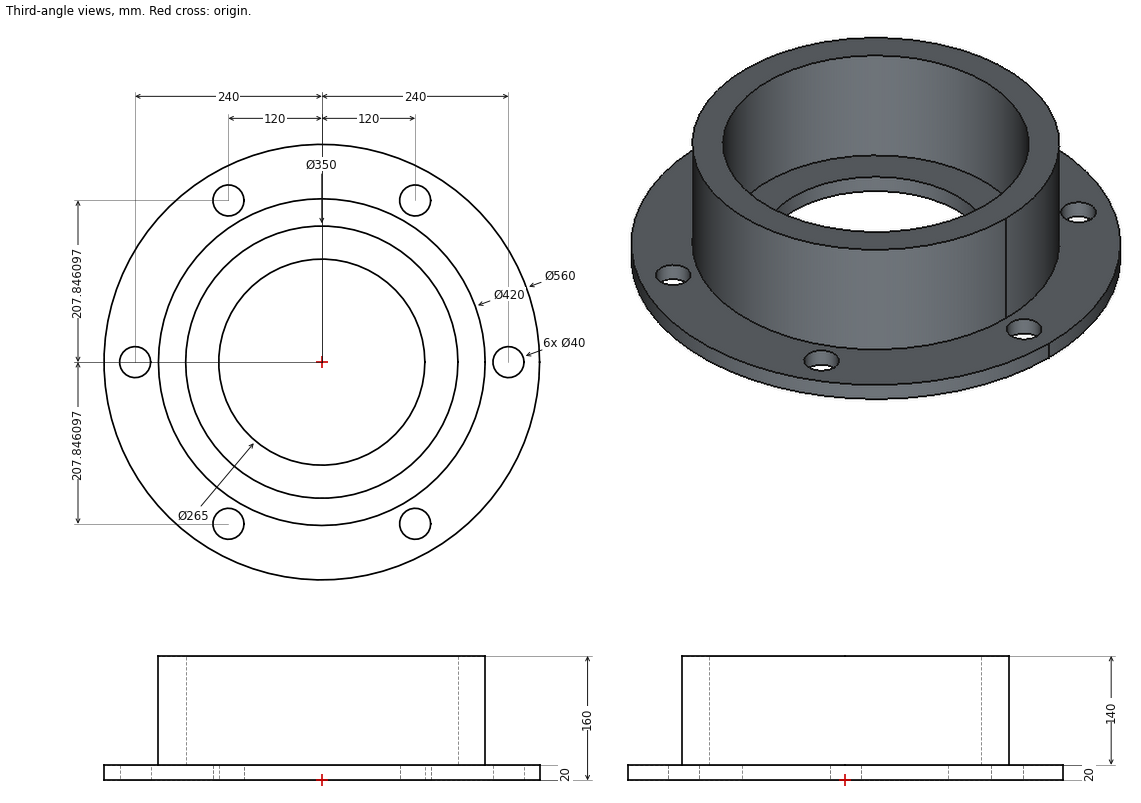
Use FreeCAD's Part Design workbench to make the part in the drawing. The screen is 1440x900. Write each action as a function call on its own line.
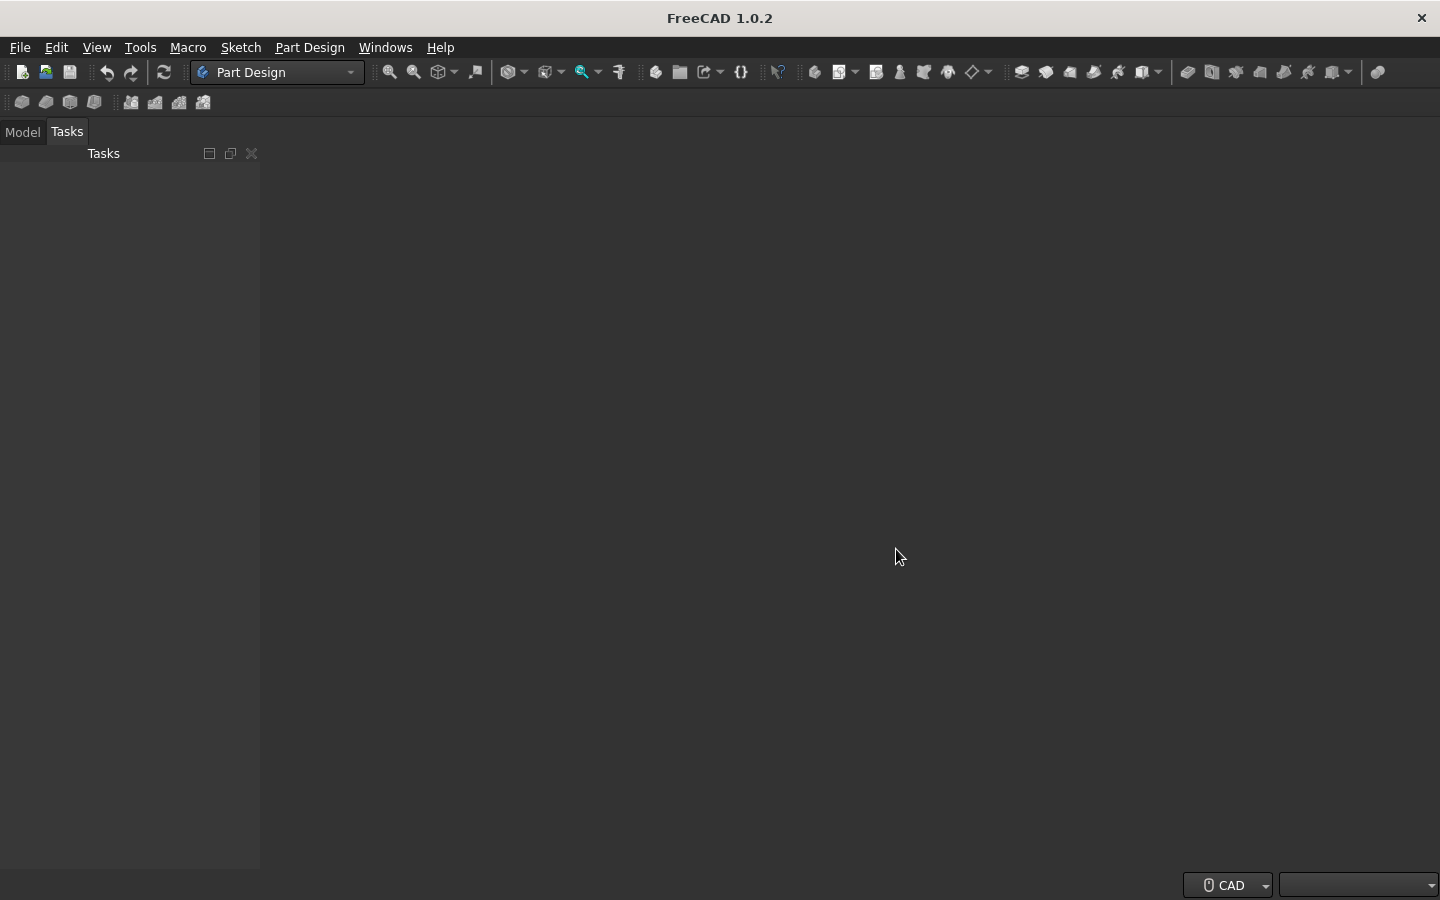
click(22, 72)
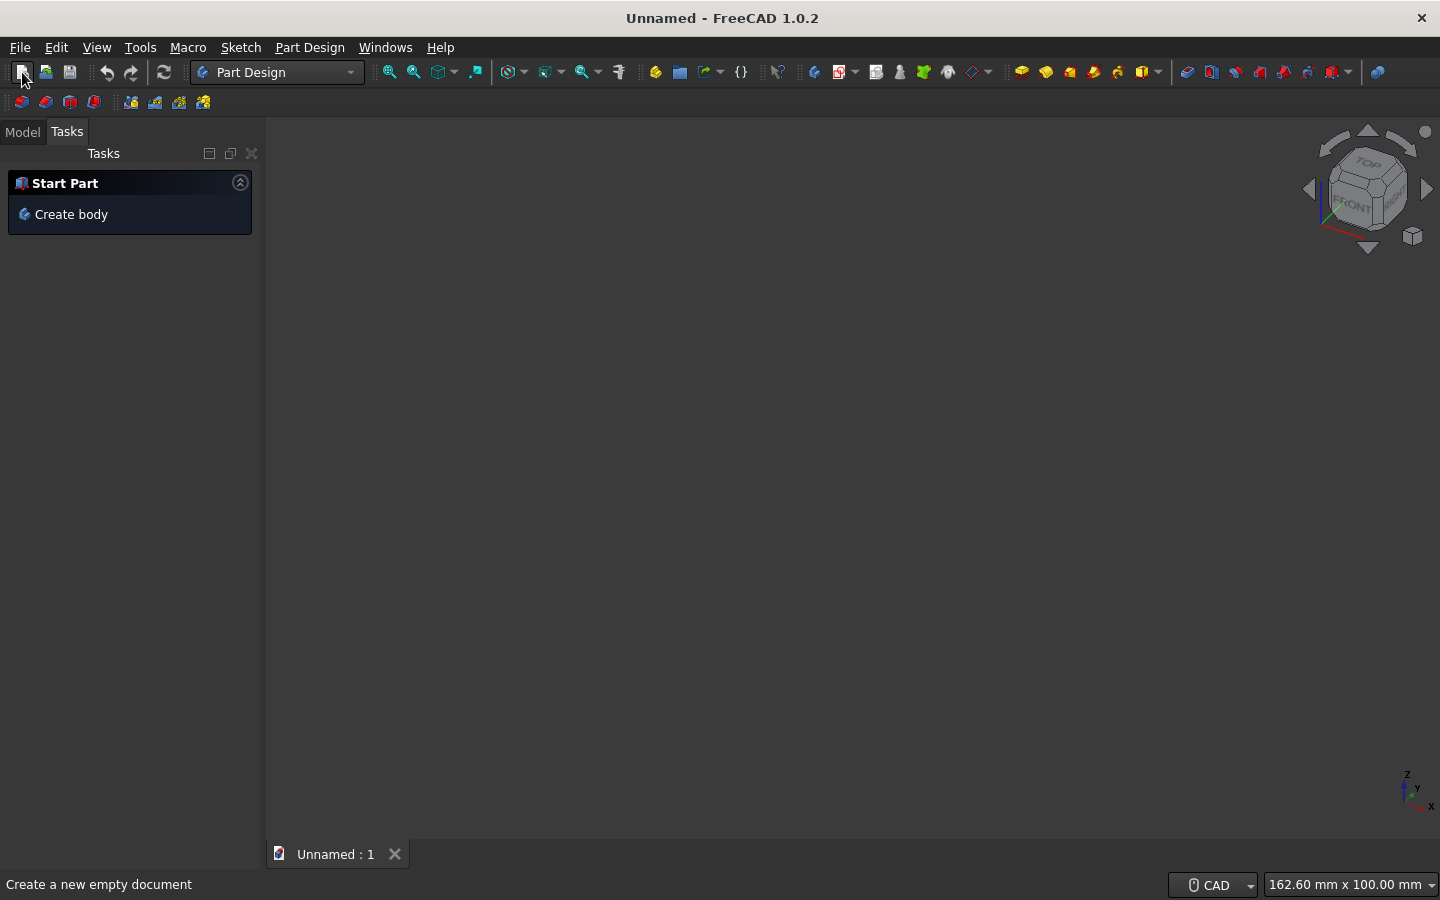
click(840, 72)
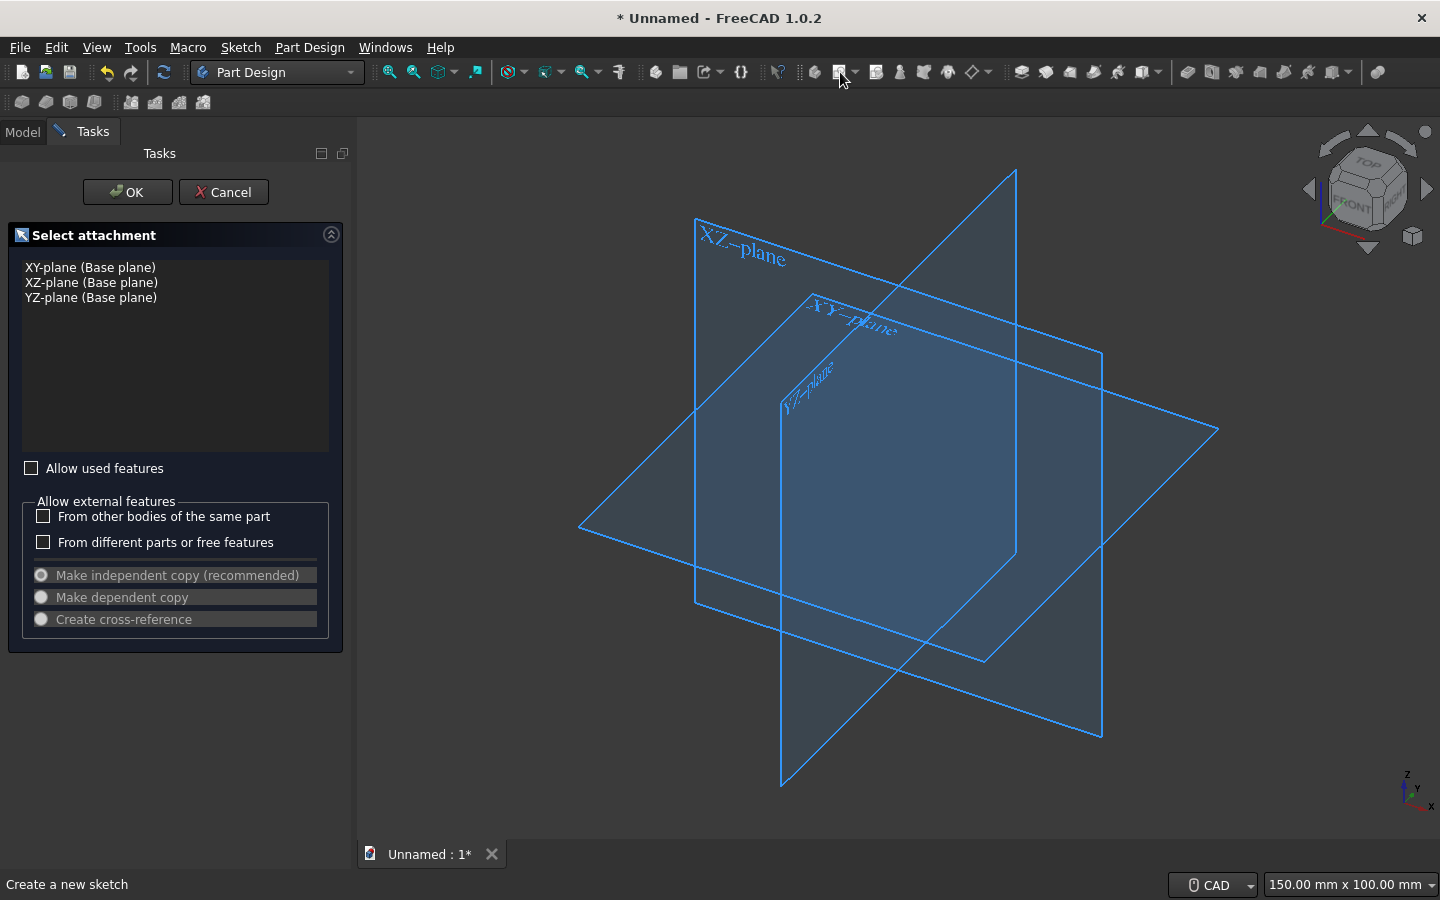
click(82, 268)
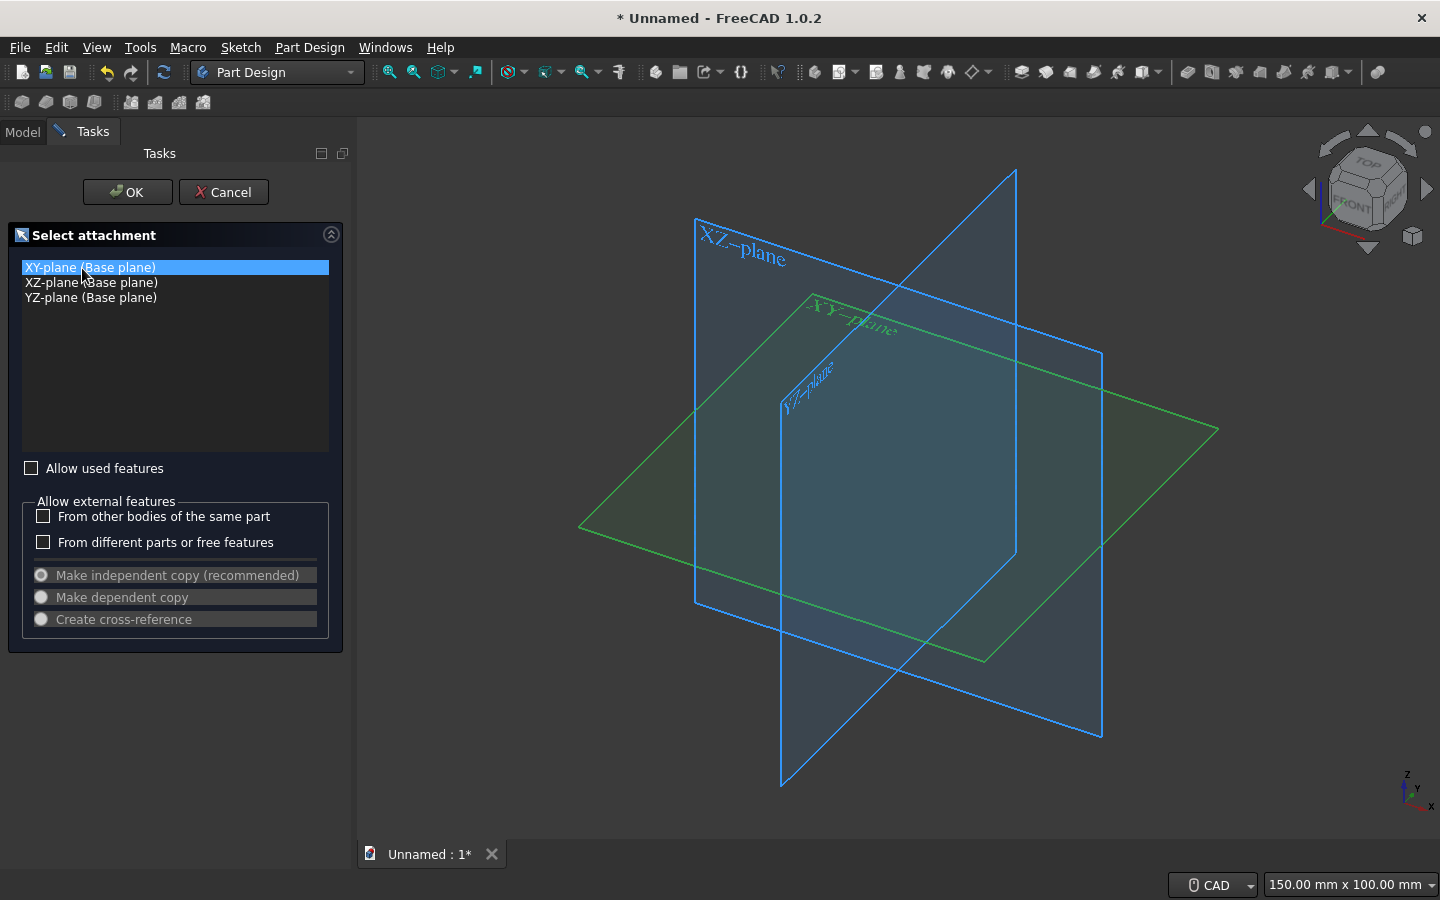
click(128, 192)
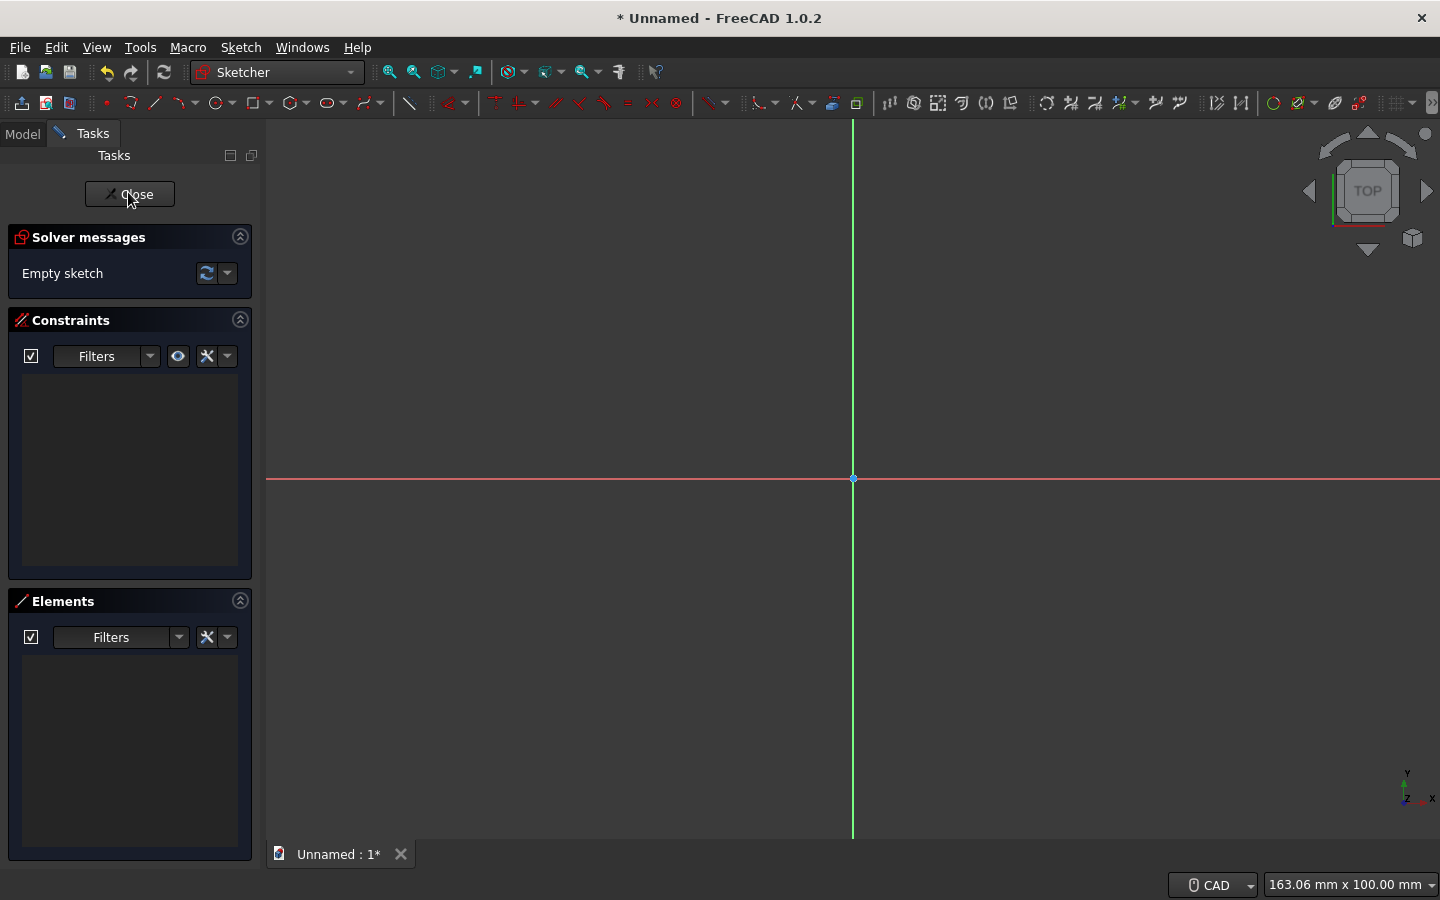
scroll(776, 479, down, 11)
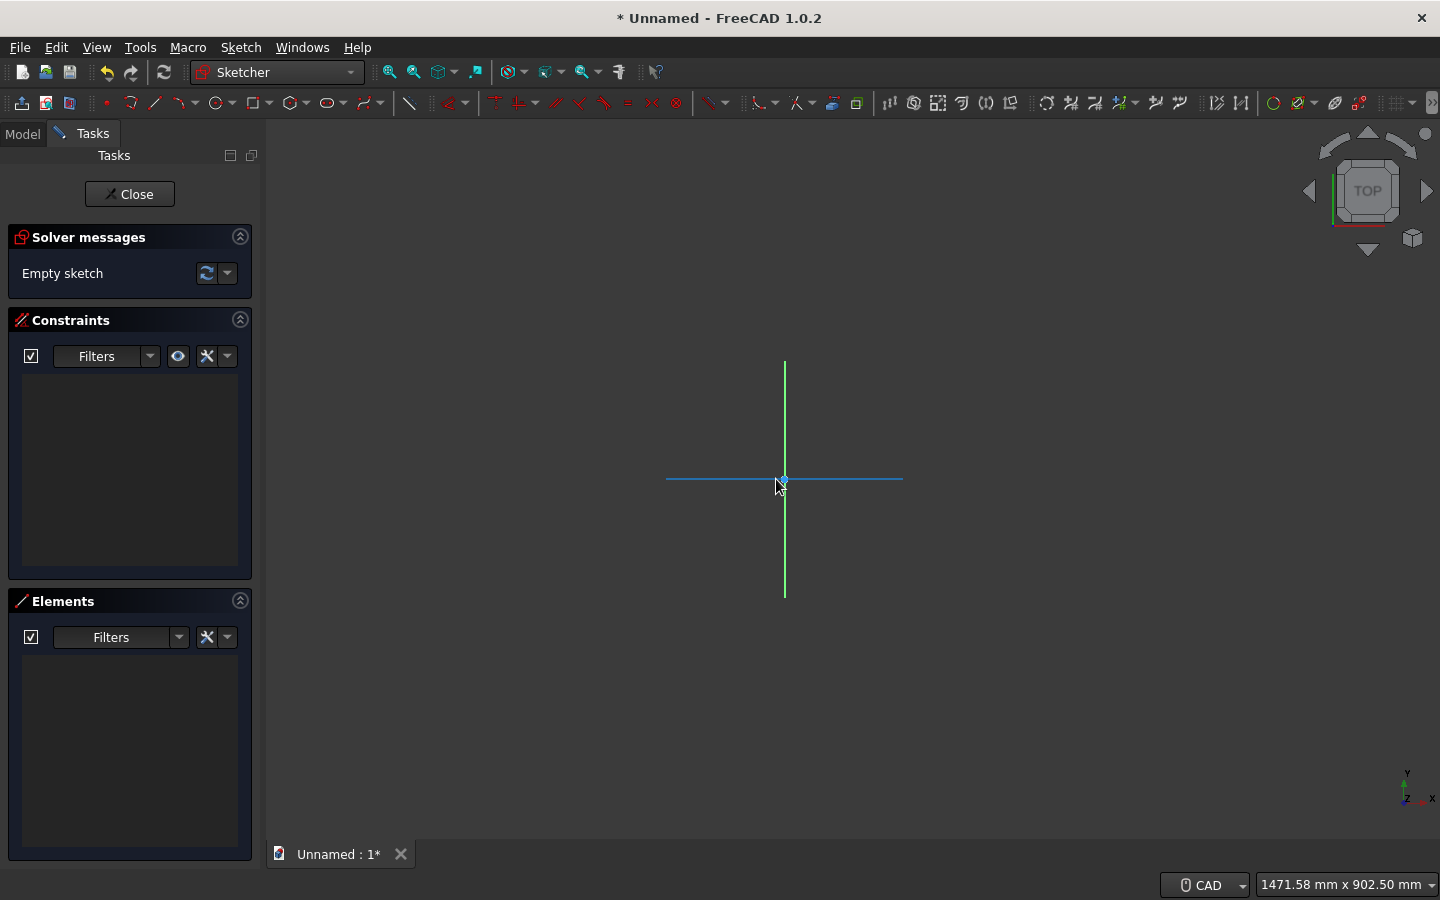
key(g)
key(c)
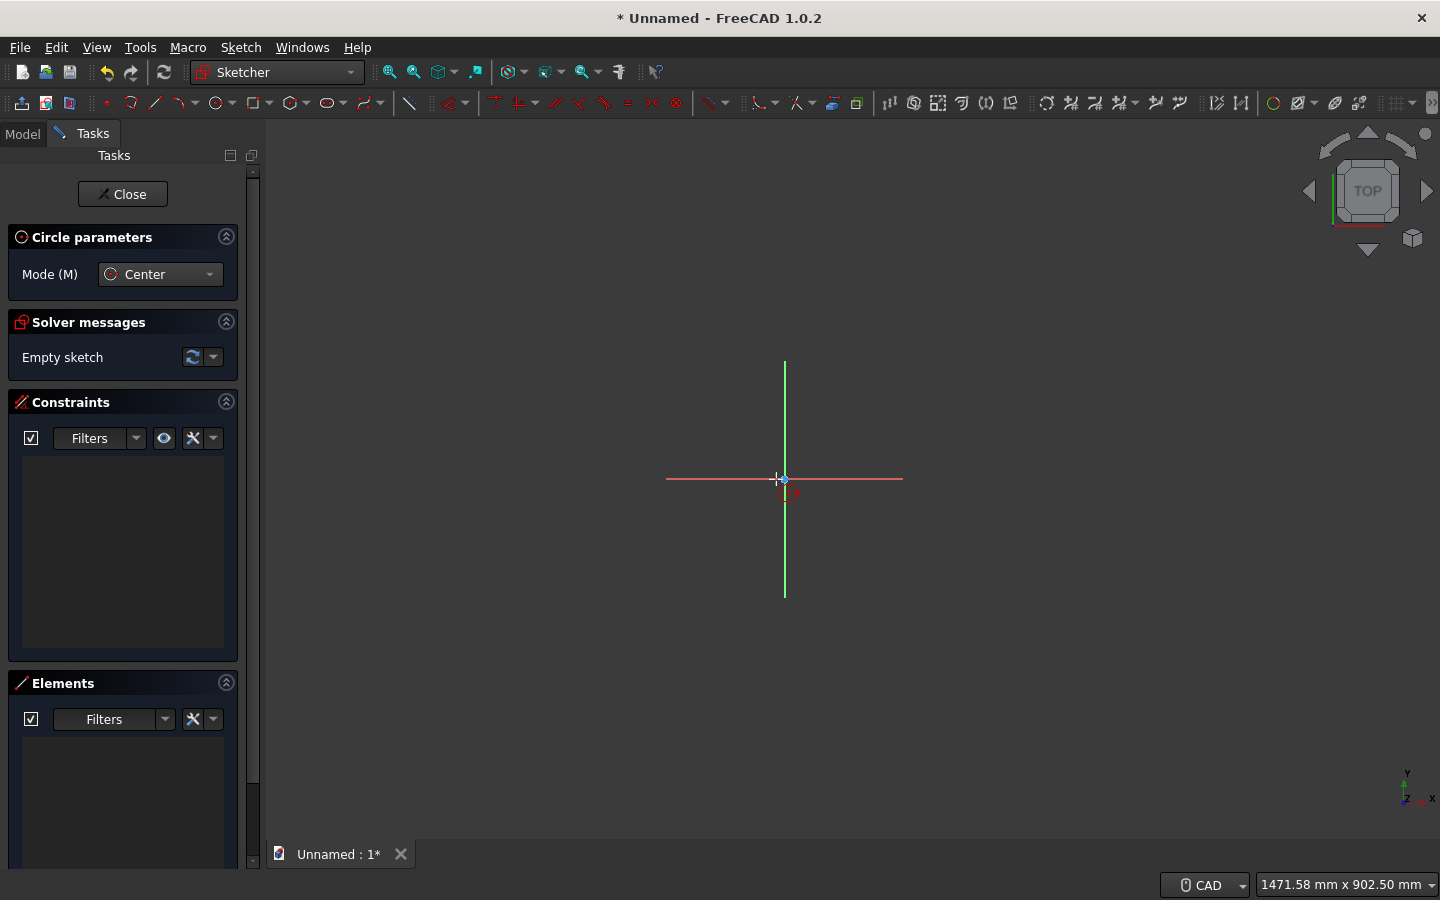
click(785, 479)
click(943, 321)
key(Escape)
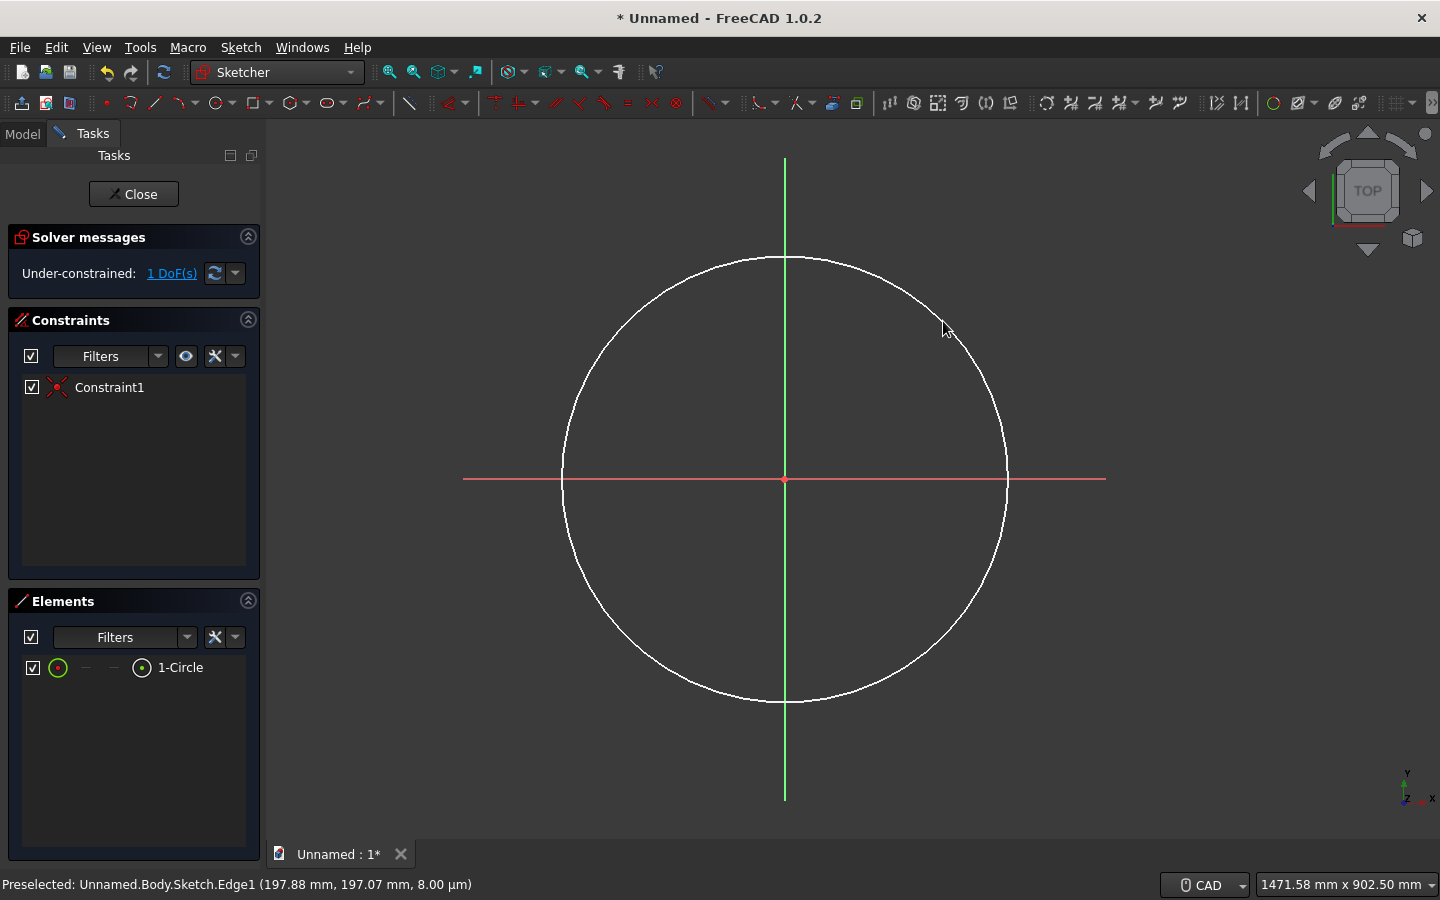
key(d)